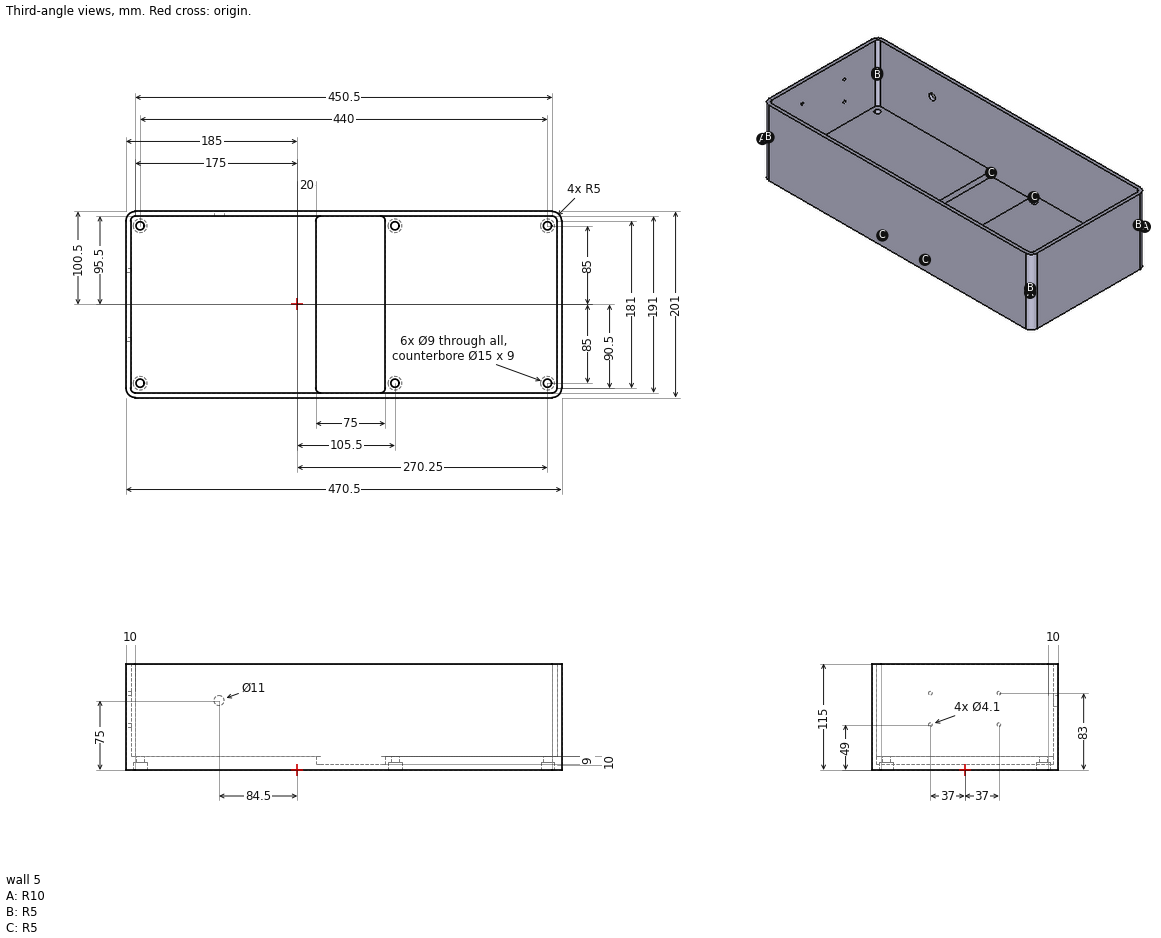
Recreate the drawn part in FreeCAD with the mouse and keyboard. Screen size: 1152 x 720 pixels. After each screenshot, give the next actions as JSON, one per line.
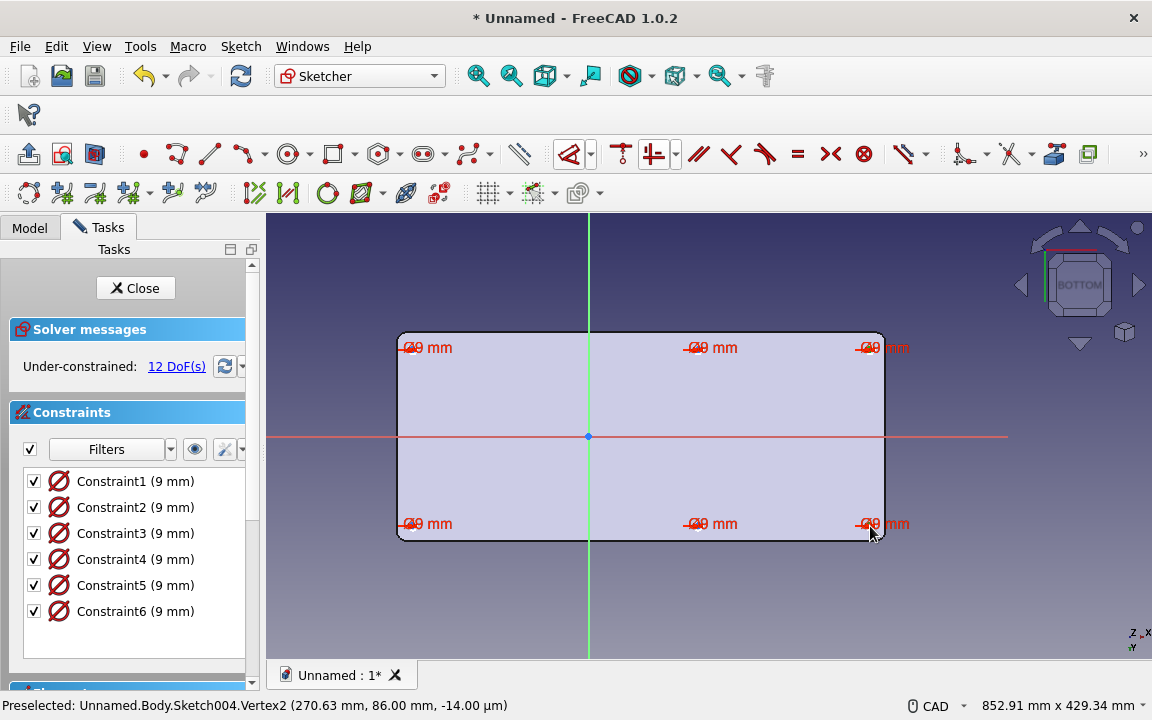
{"action": "key", "text": "v"}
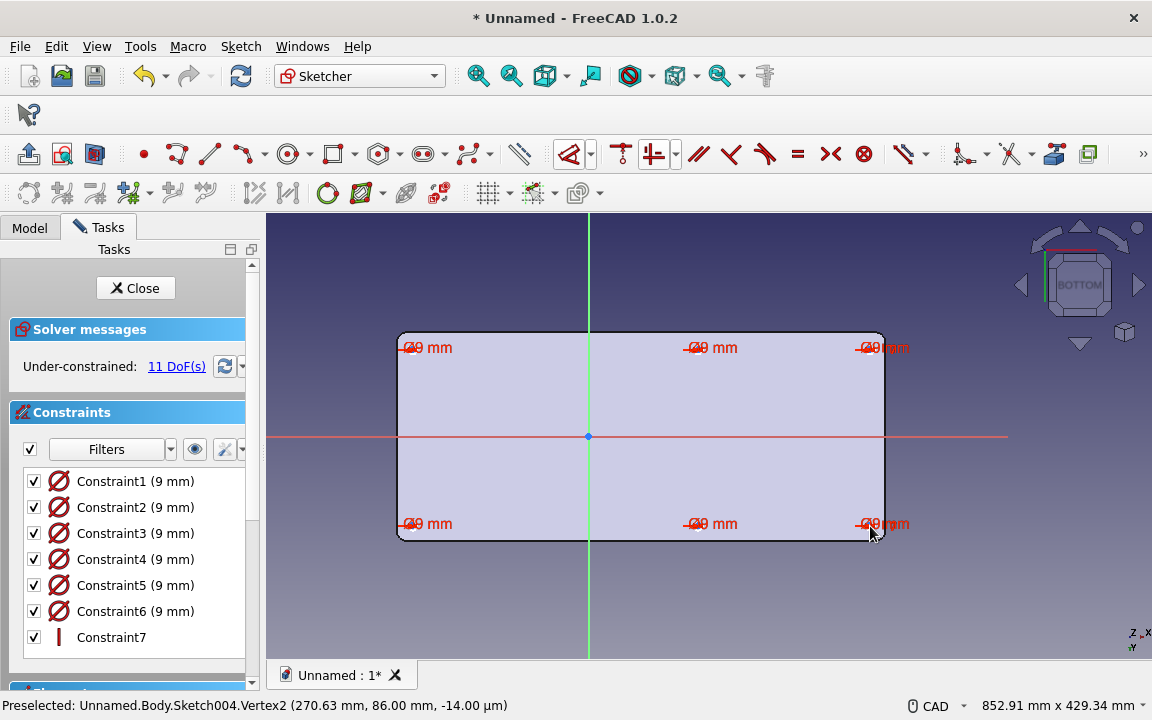
{"action": "left_click", "coordinate": [870, 526]}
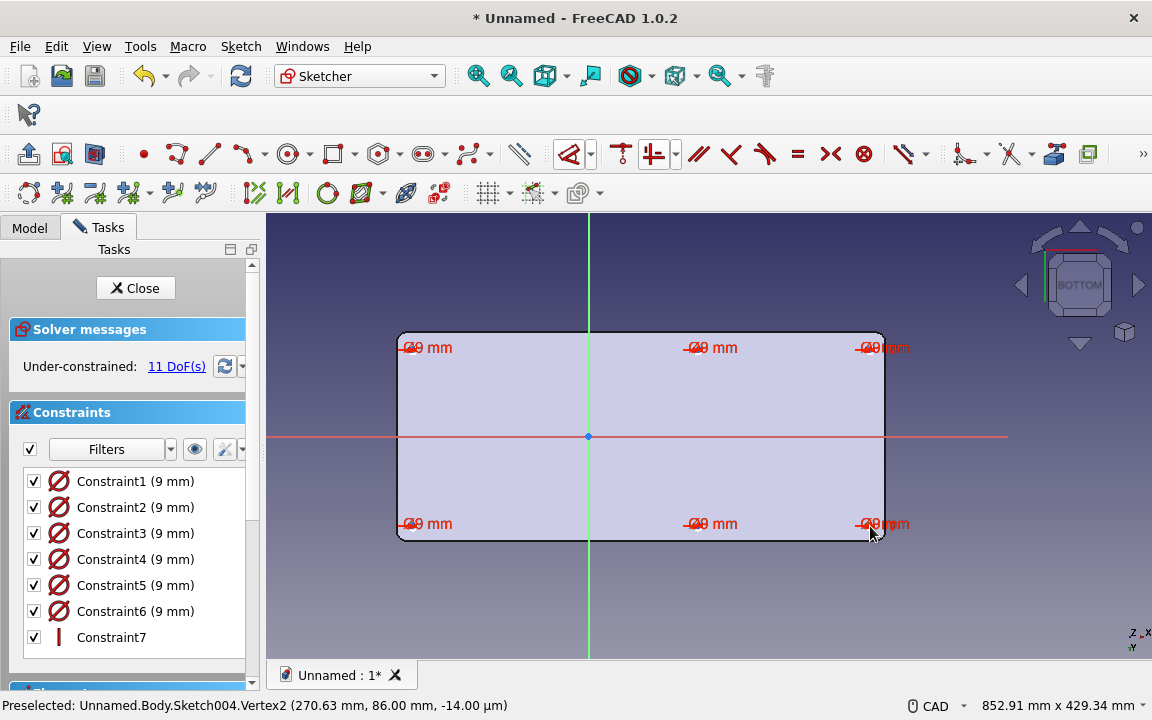
{"action": "left_click", "coordinate": [413, 526]}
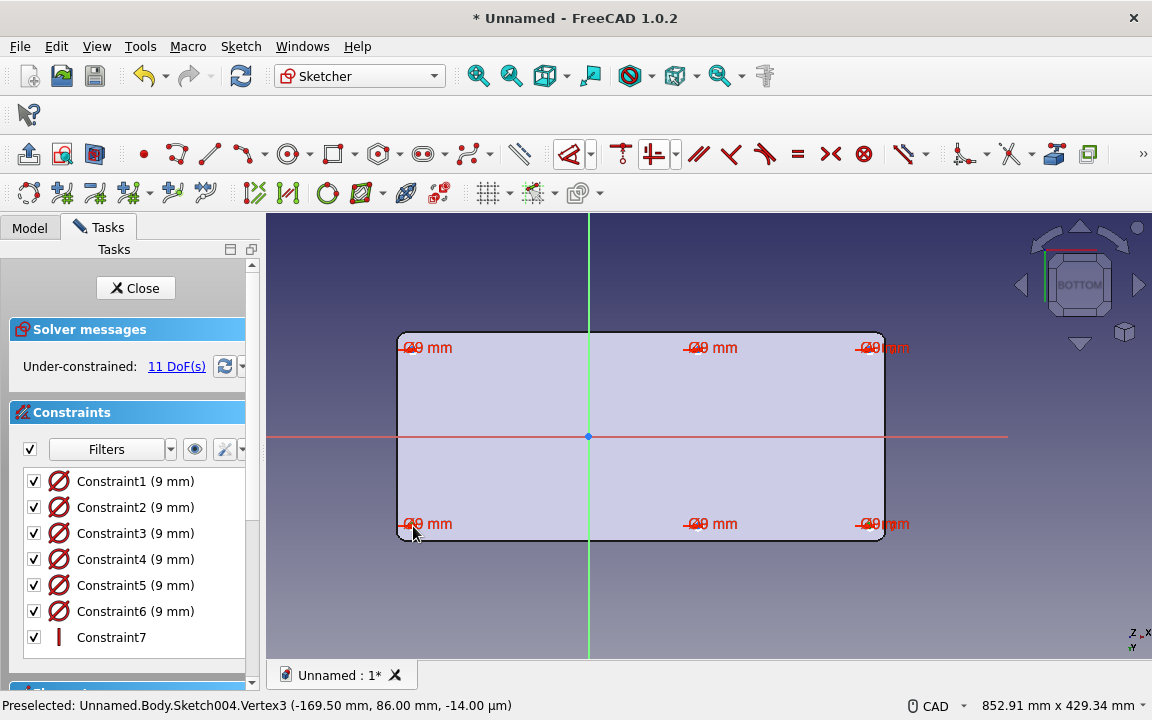
{"action": "key", "text": "h"}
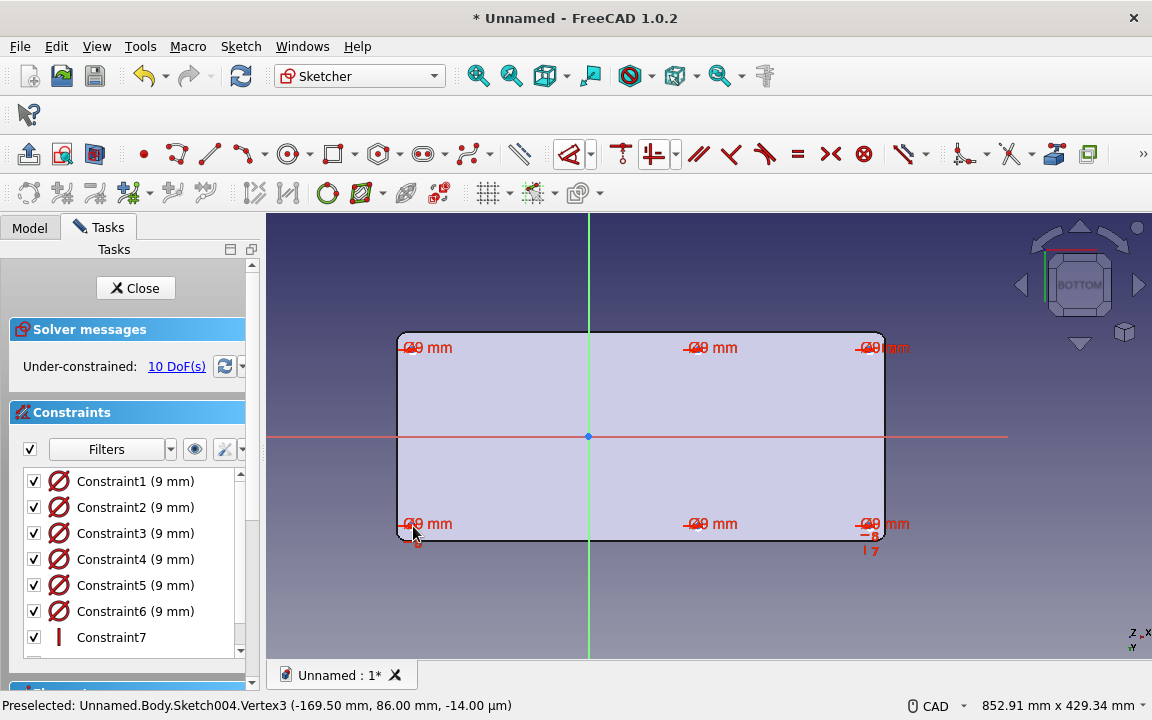
{"action": "left_click", "coordinate": [413, 526]}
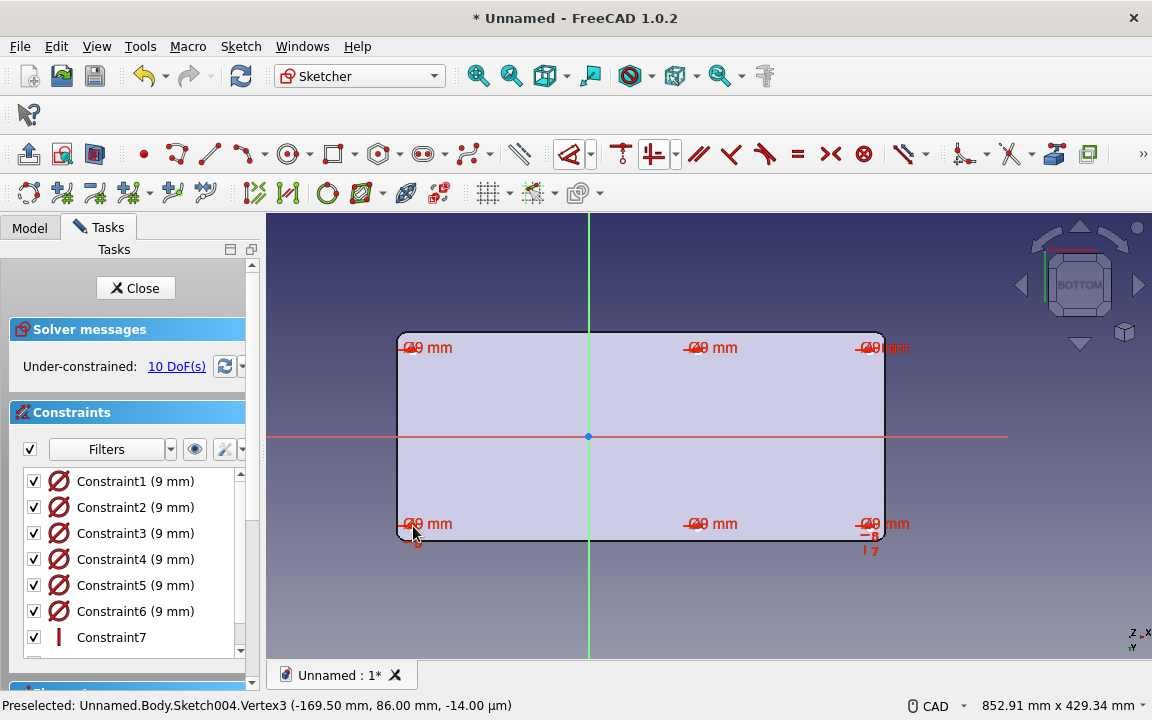
{"action": "left_click", "coordinate": [413, 350]}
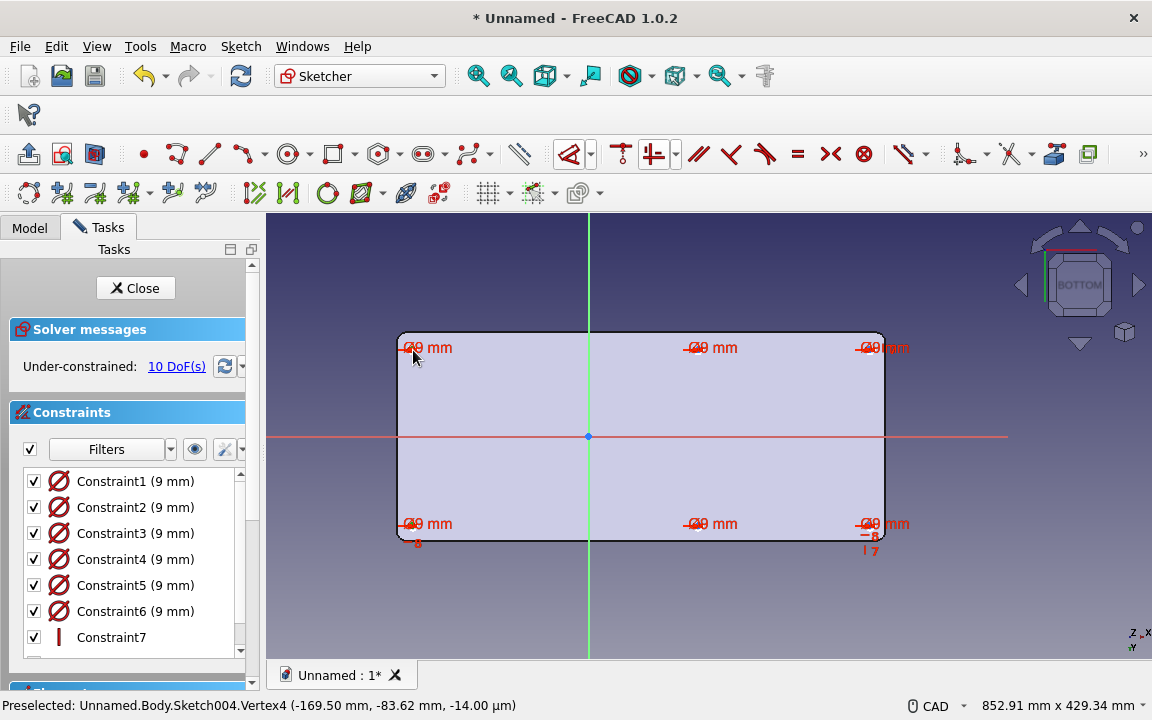
{"action": "key", "text": "v"}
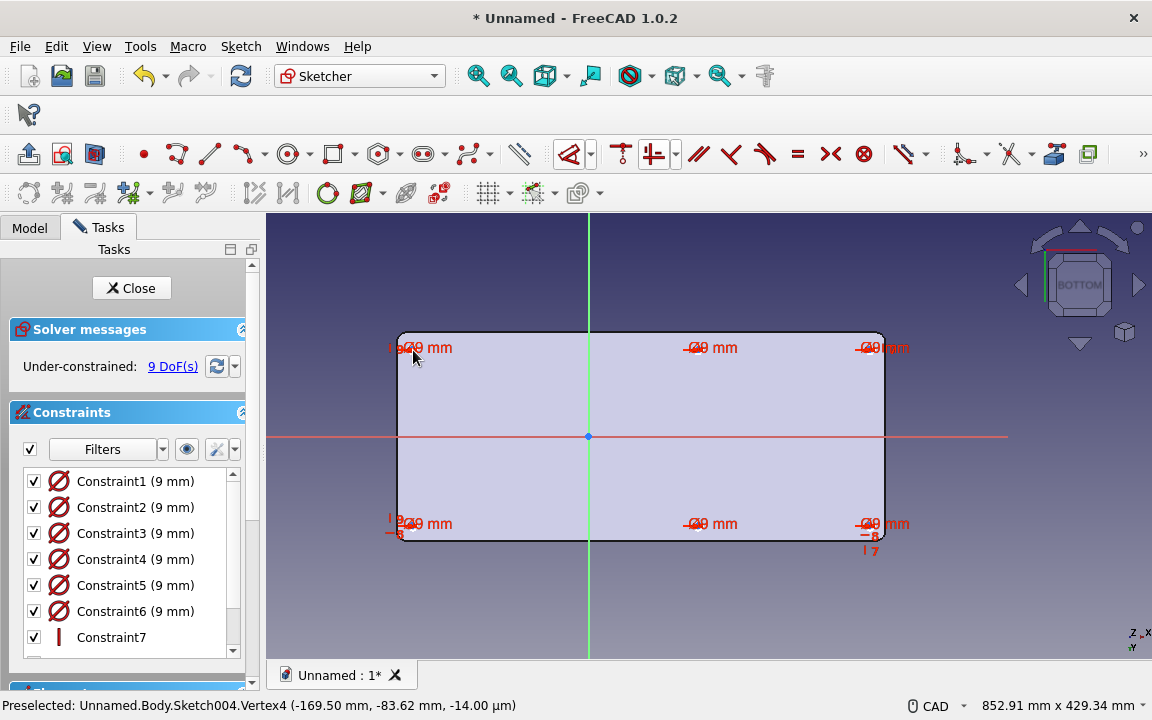
{"action": "left_click", "coordinate": [870, 350]}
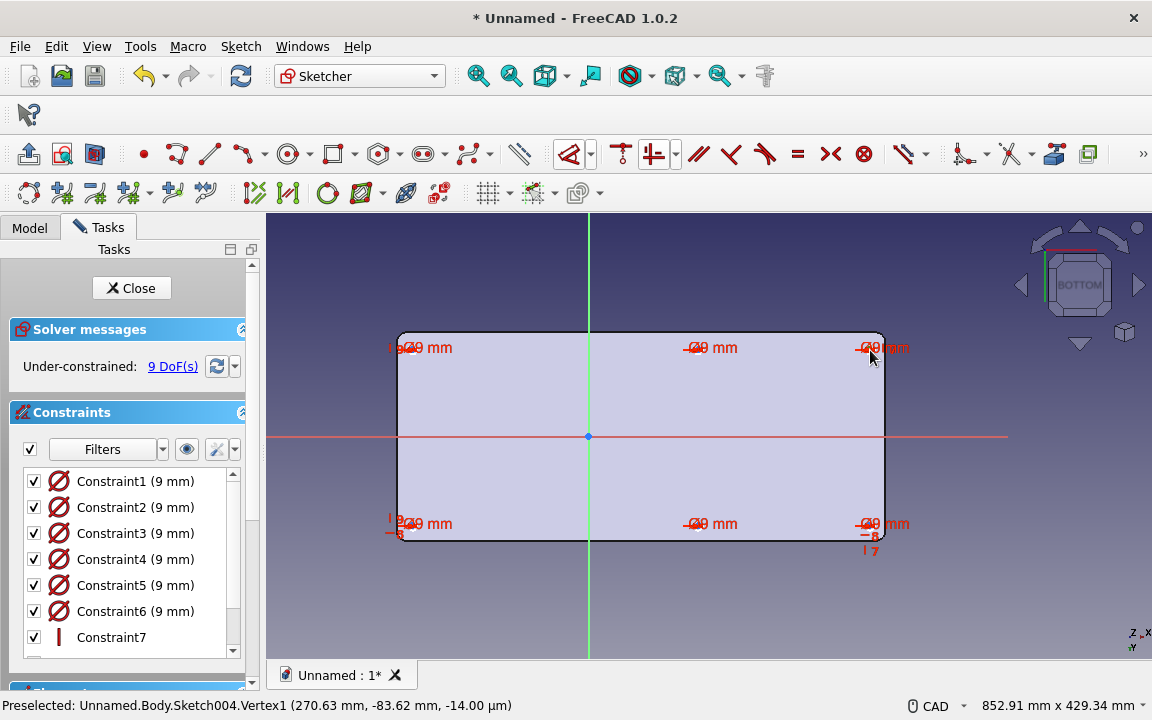
{"action": "left_click", "coordinate": [413, 350]}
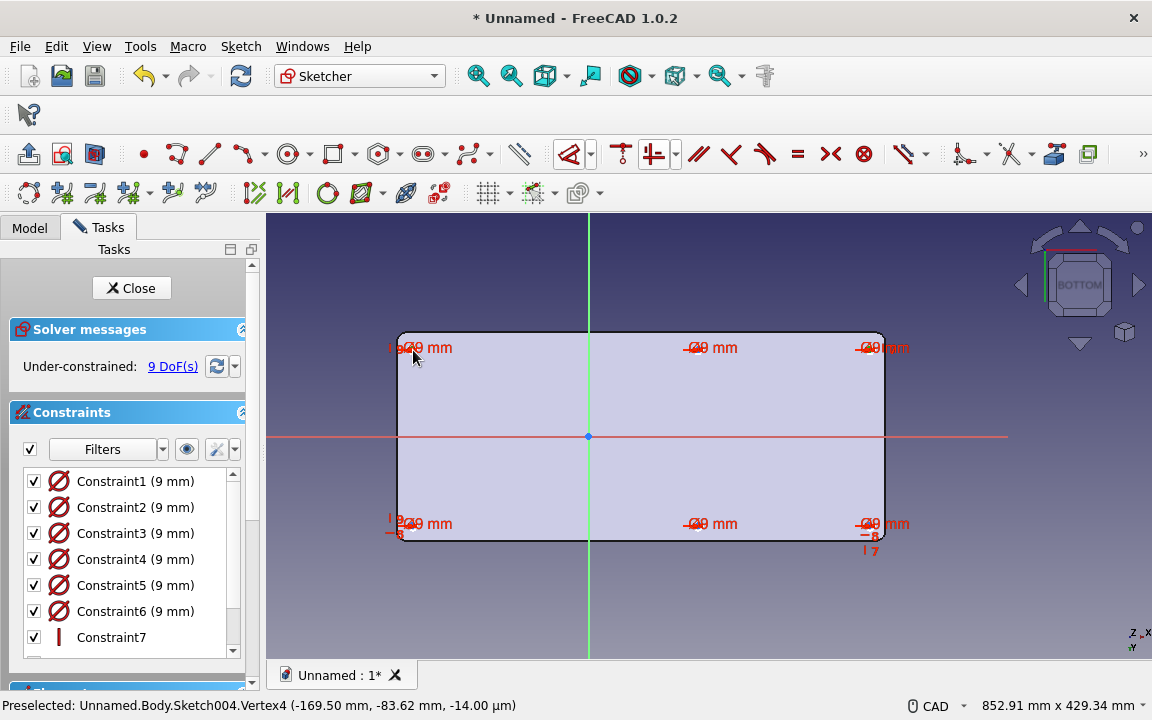
{"action": "left_click", "coordinate": [676, 154]}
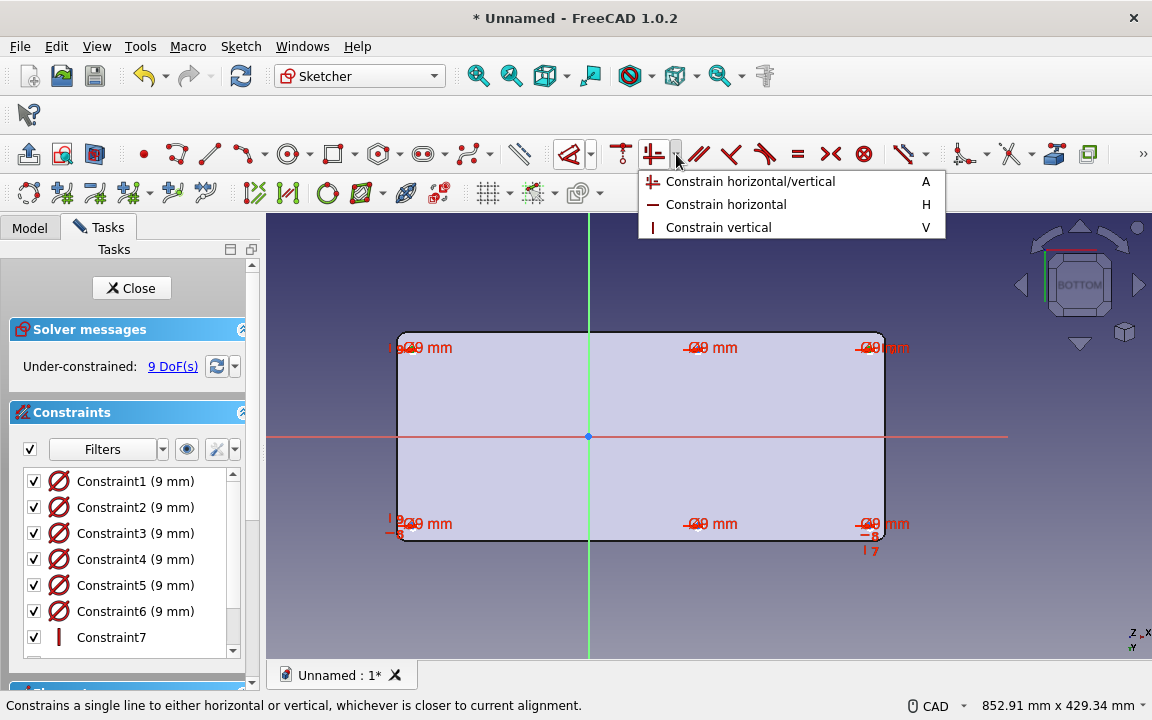
{"action": "left_click", "coordinate": [792, 204]}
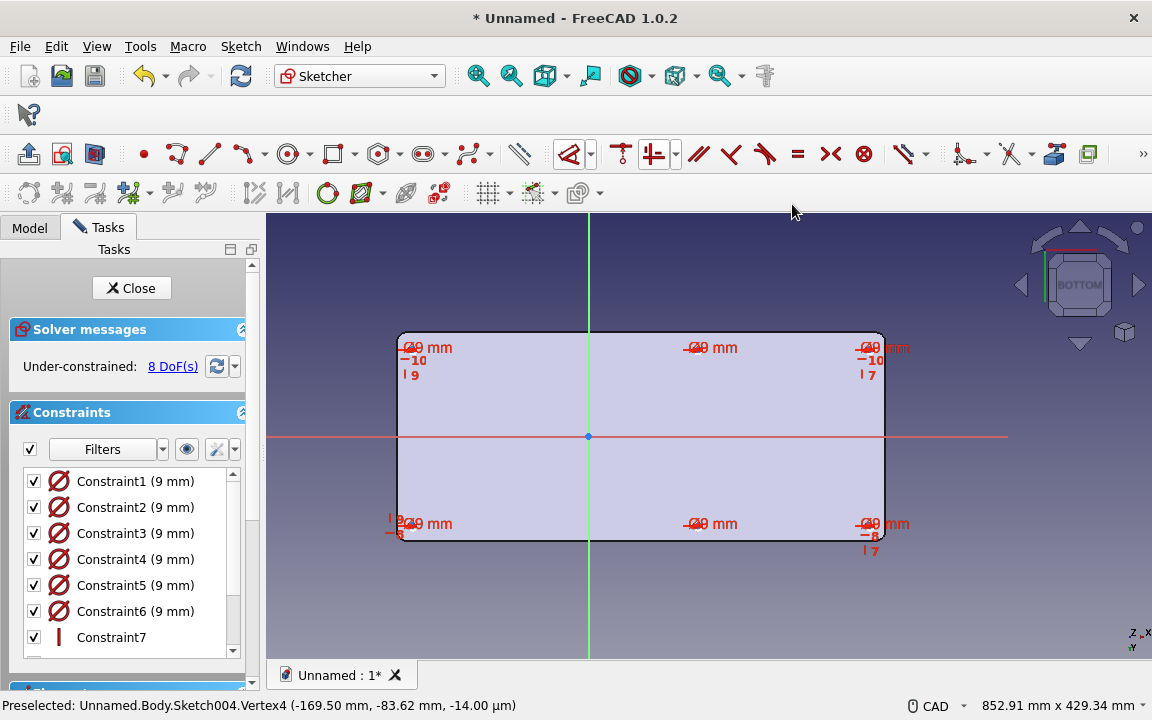
{"action": "left_click", "coordinate": [870, 350]}